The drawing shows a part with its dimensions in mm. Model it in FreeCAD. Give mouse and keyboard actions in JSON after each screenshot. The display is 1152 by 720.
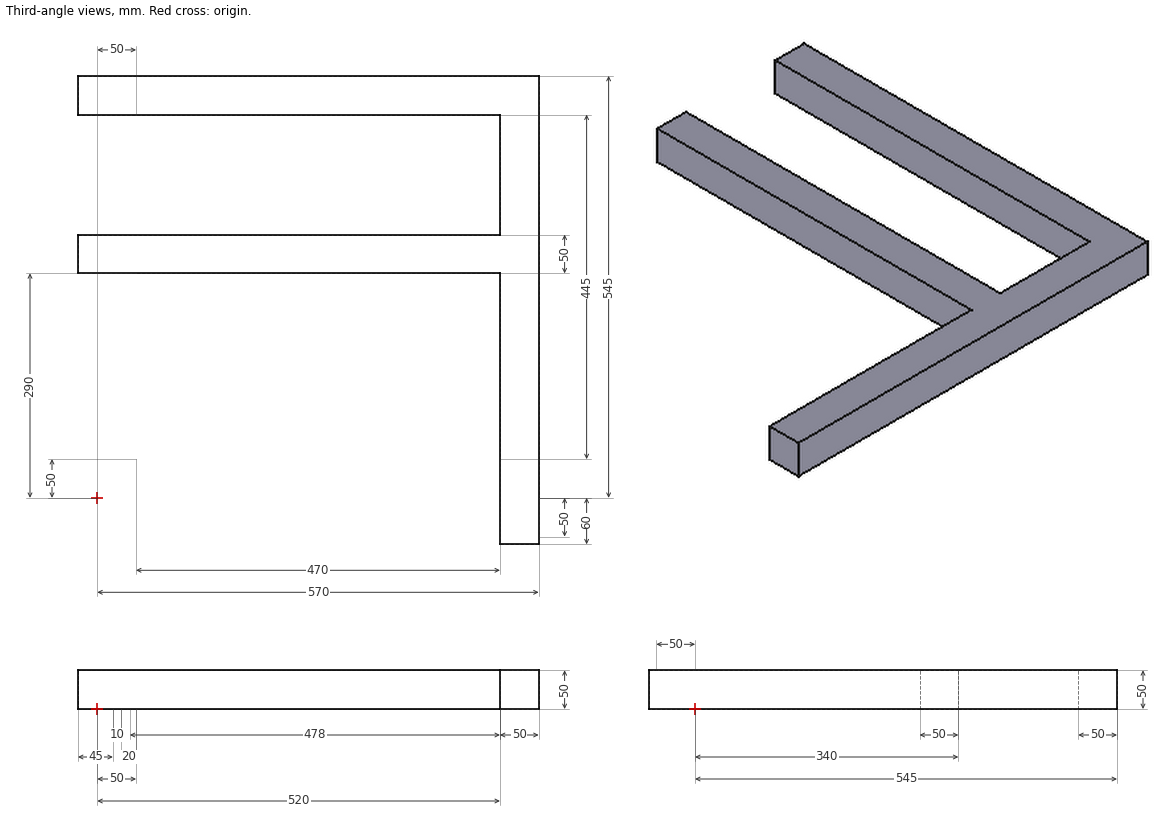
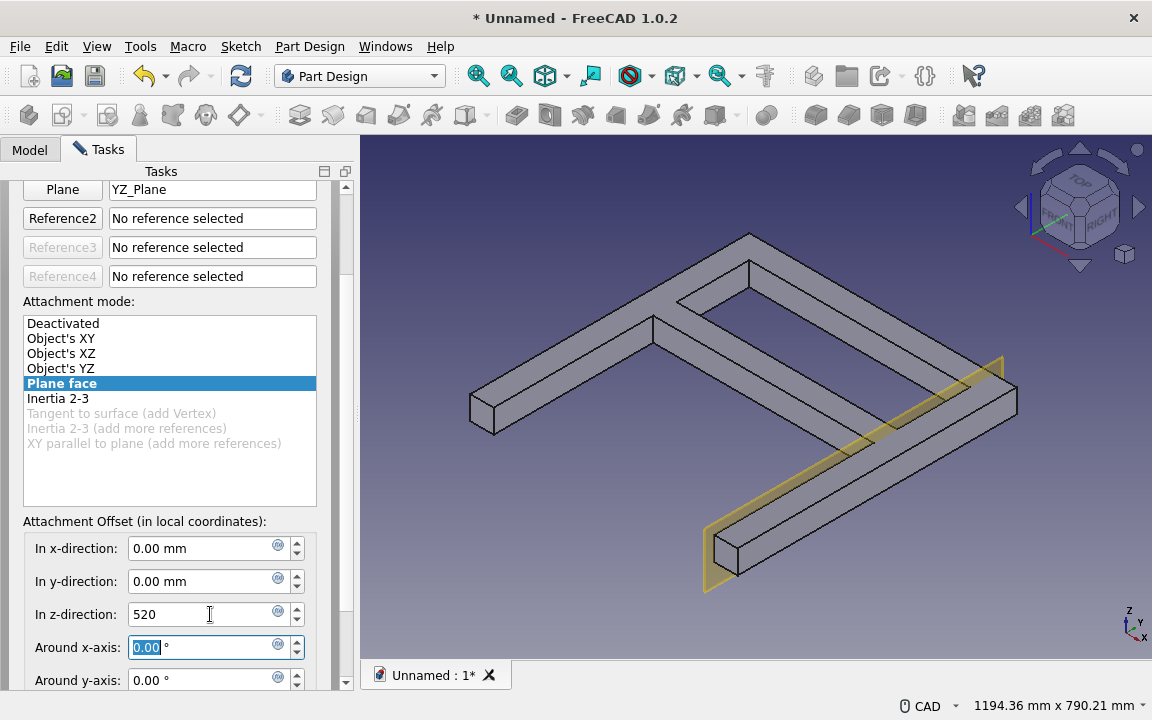
{"action": "scroll", "coordinate": [346, 436], "scroll_direction": "up", "scroll_amount": 3}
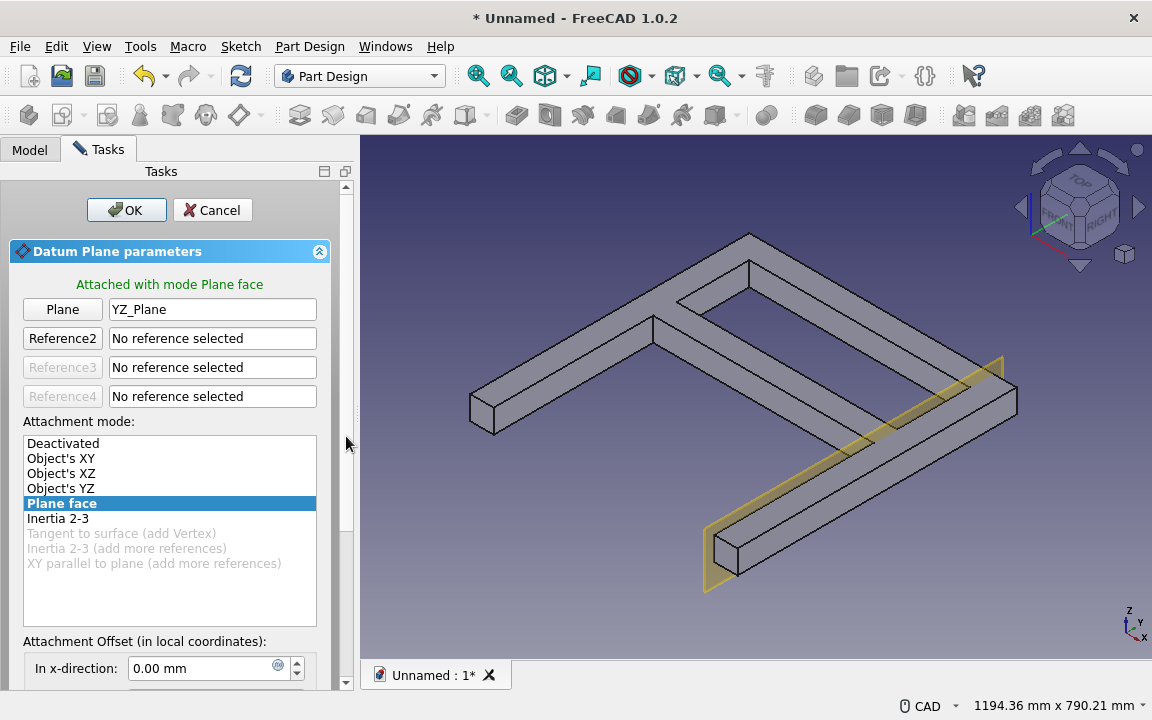
{"action": "left_click", "coordinate": [127, 210]}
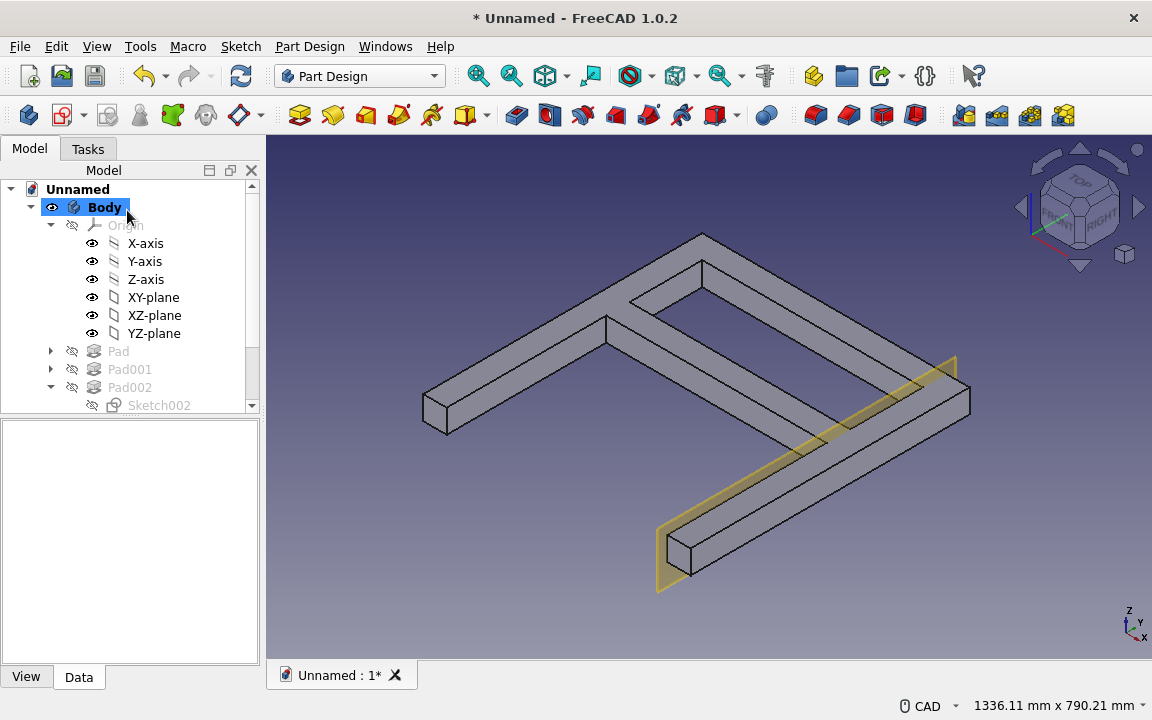
{"action": "scroll", "coordinate": [101, 293], "scroll_direction": "down", "scroll_amount": 3}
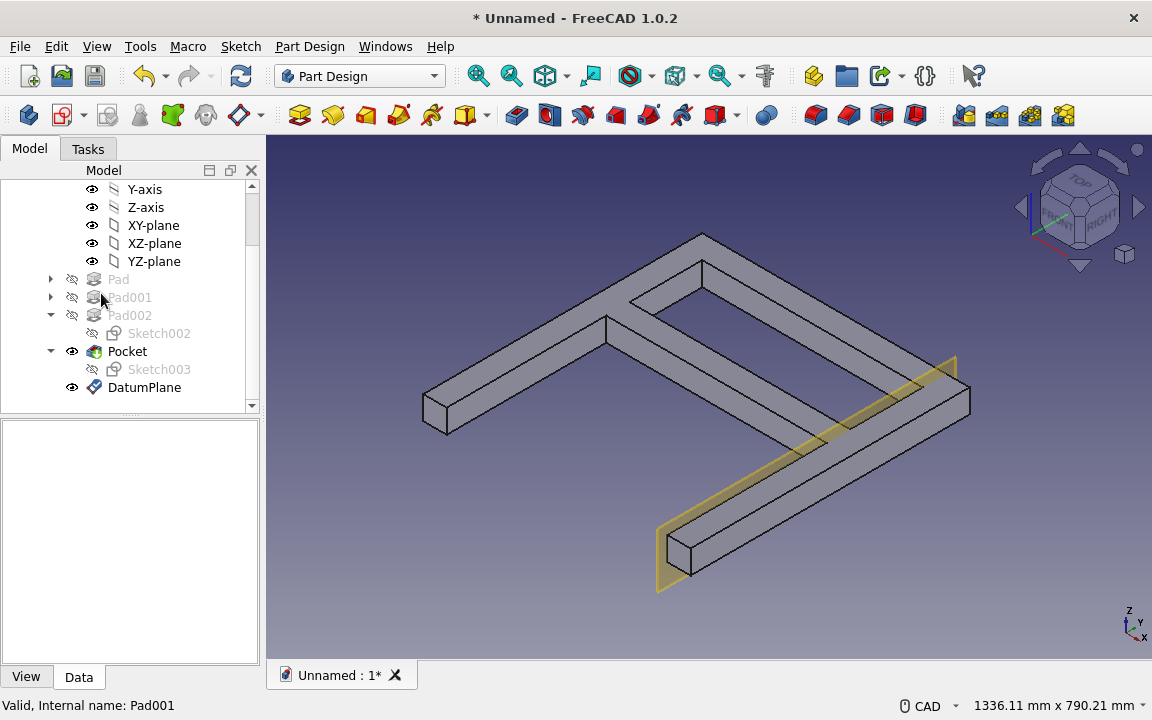
{"action": "left_click", "coordinate": [117, 387]}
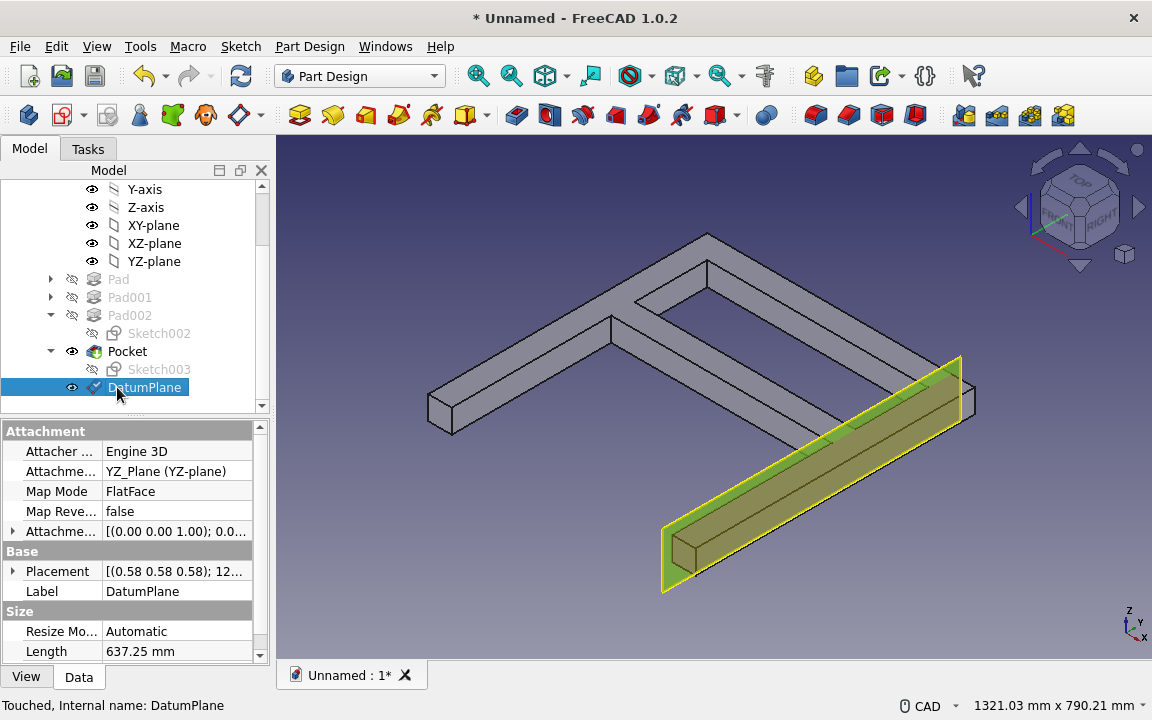
{"action": "left_click", "coordinate": [62, 116]}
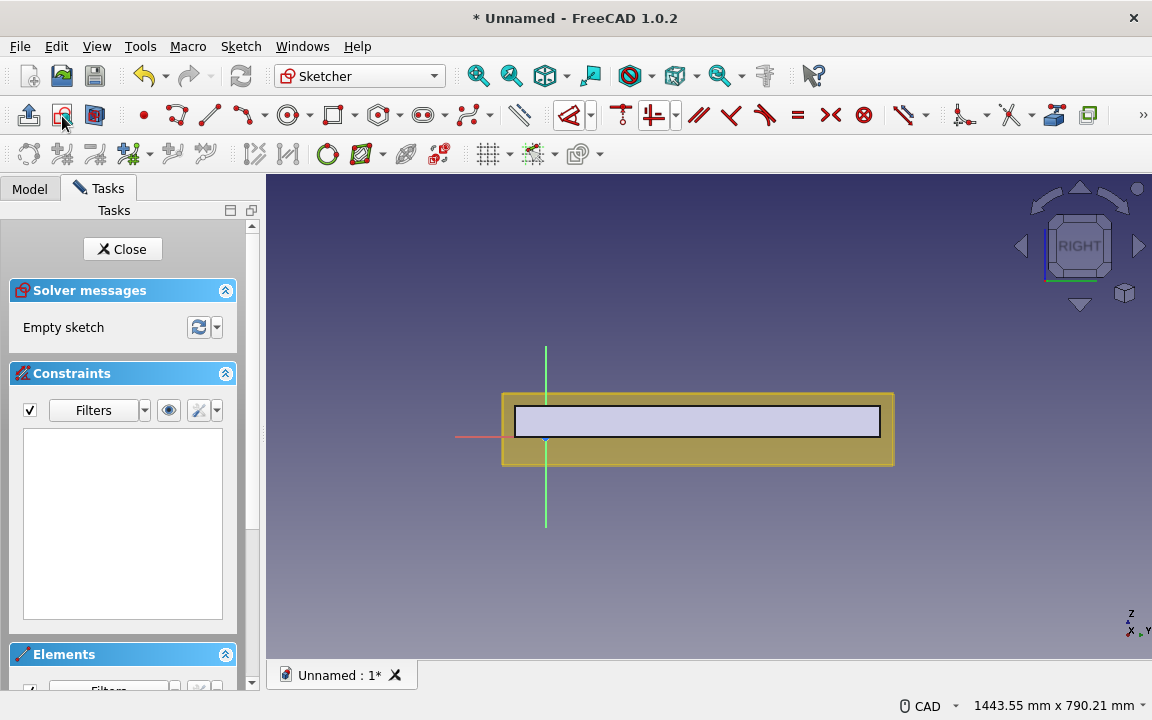
{"action": "key", "text": "q s"}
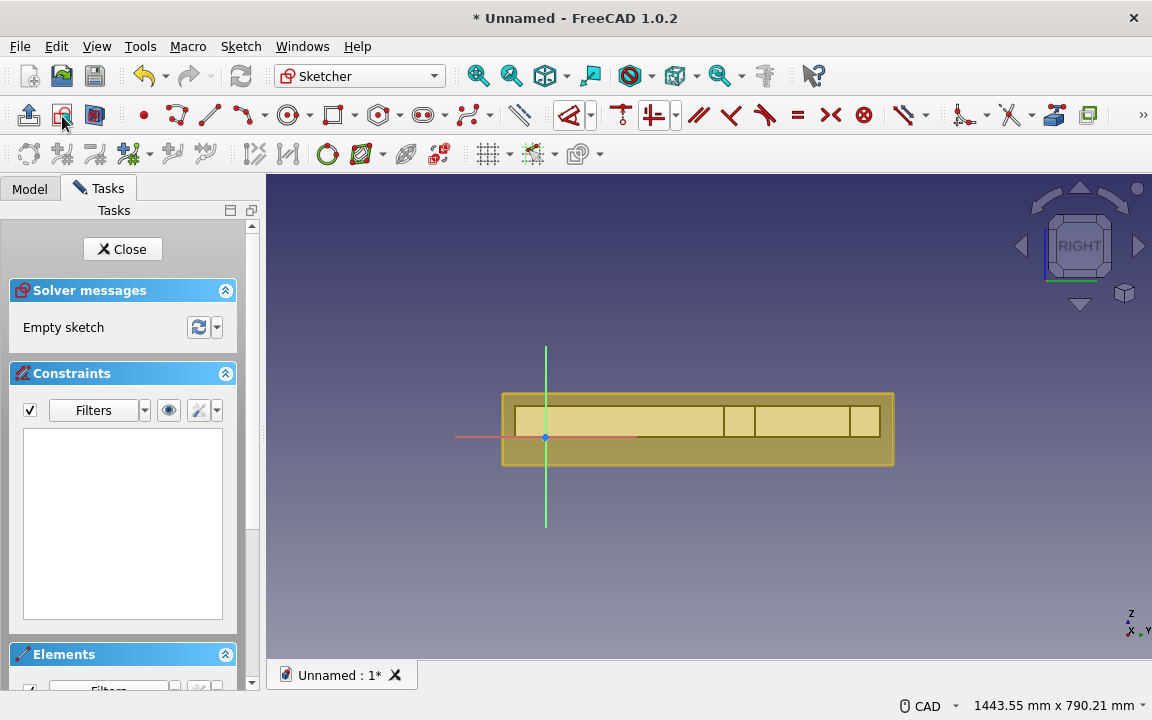
{"action": "scroll", "coordinate": [517, 422], "scroll_direction": "up", "scroll_amount": 11}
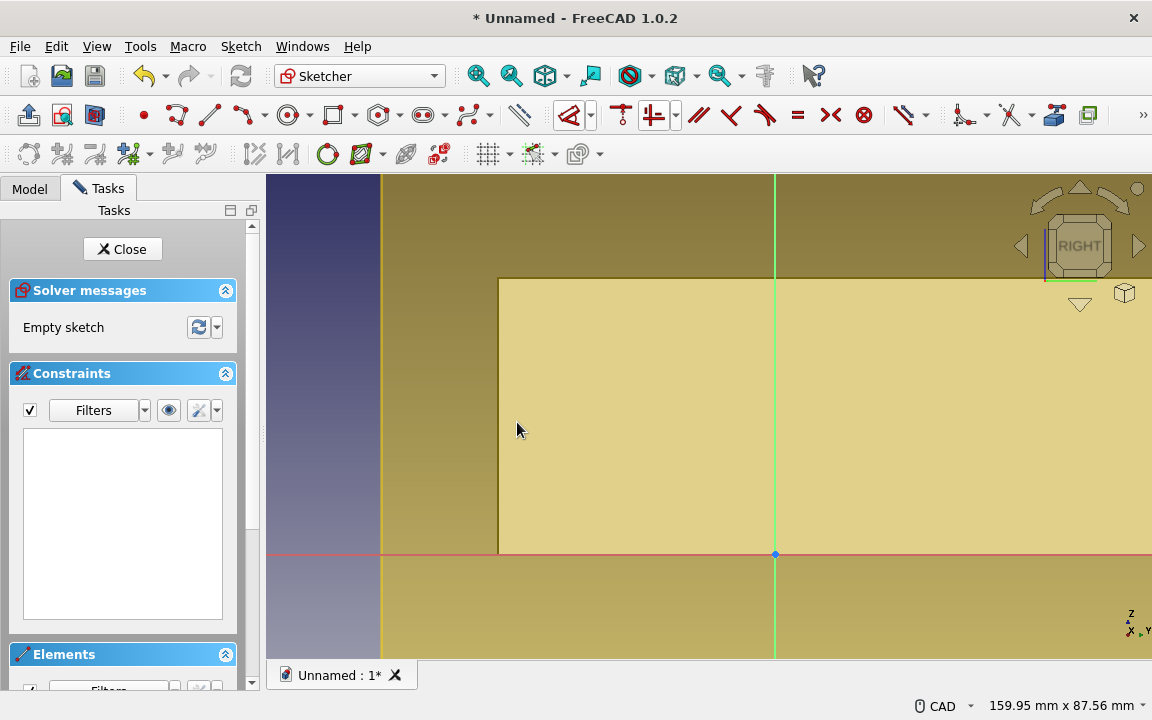
{"action": "key", "text": "g r"}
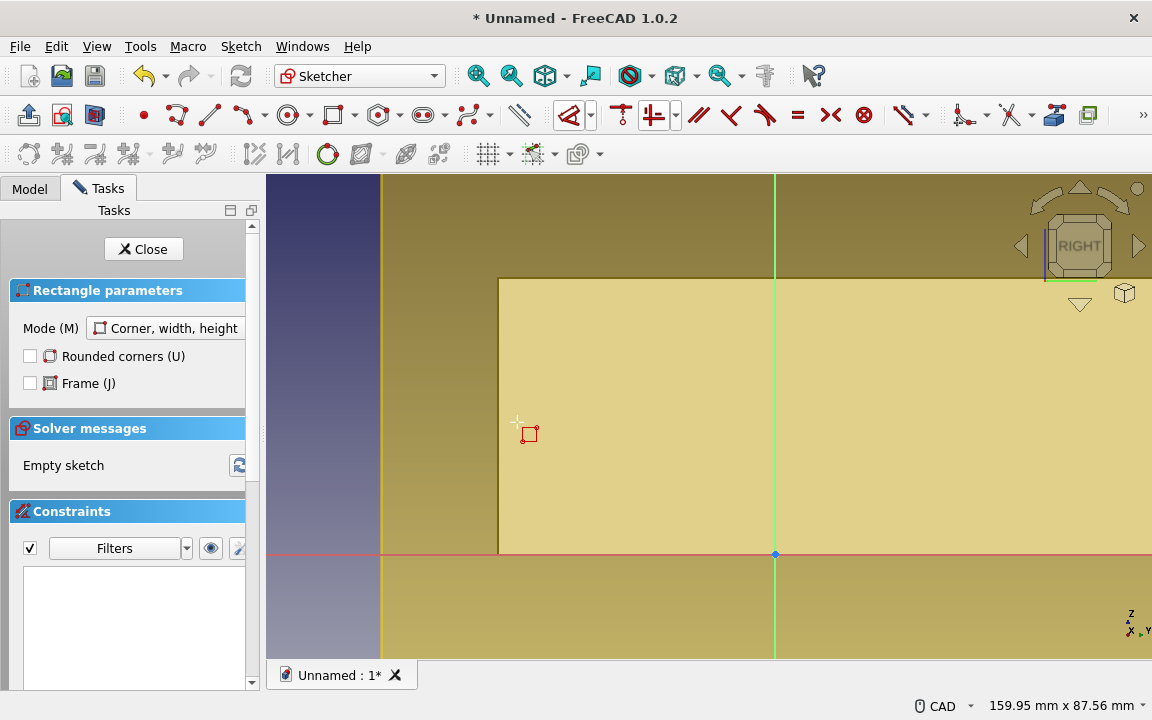
{"action": "left_click", "coordinate": [775, 555]}
{"action": "mouse_move", "coordinate": [498, 278]}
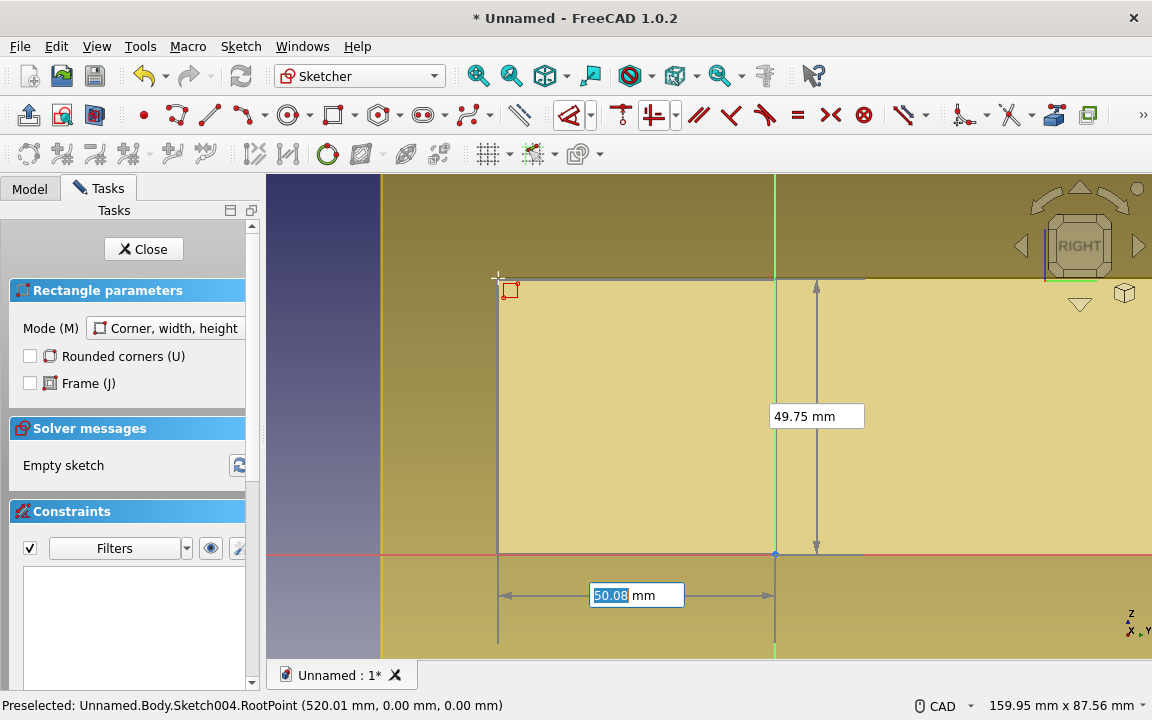
{"action": "type", "text": "50"}
{"action": "key", "text": "Tab"}
{"action": "type", "text": "50"}
{"action": "key", "text": "Return"}
{"action": "key", "text": "Escape"}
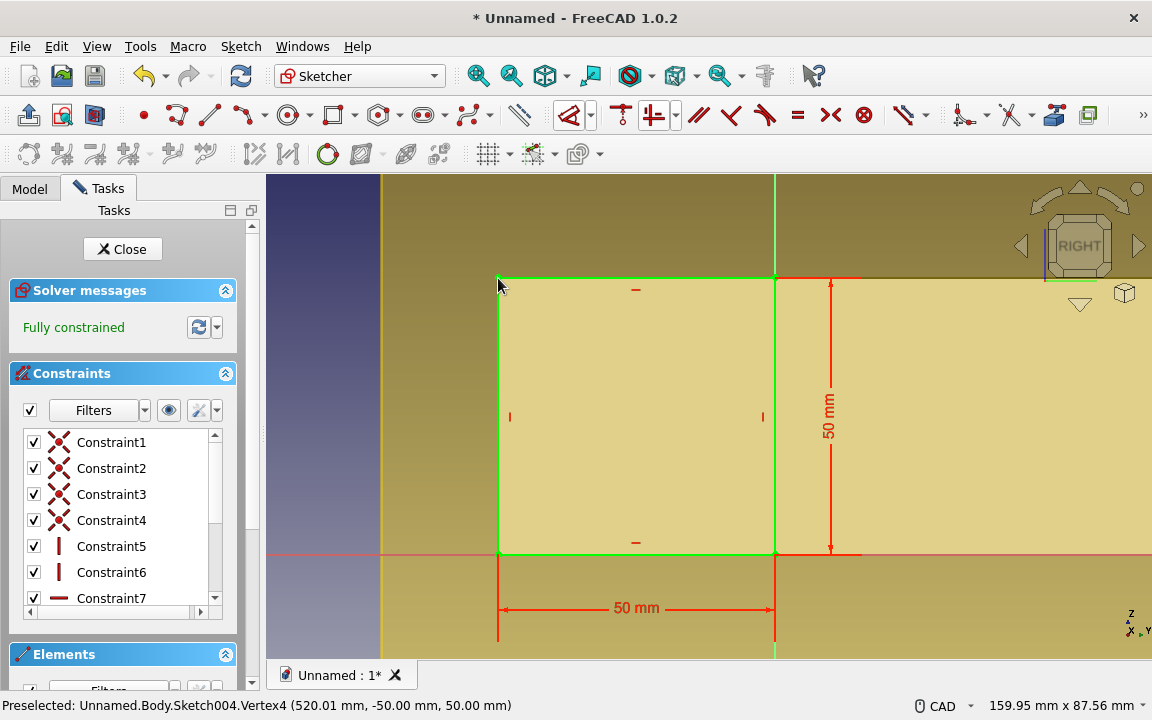
{"action": "left_click", "coordinate": [123, 249]}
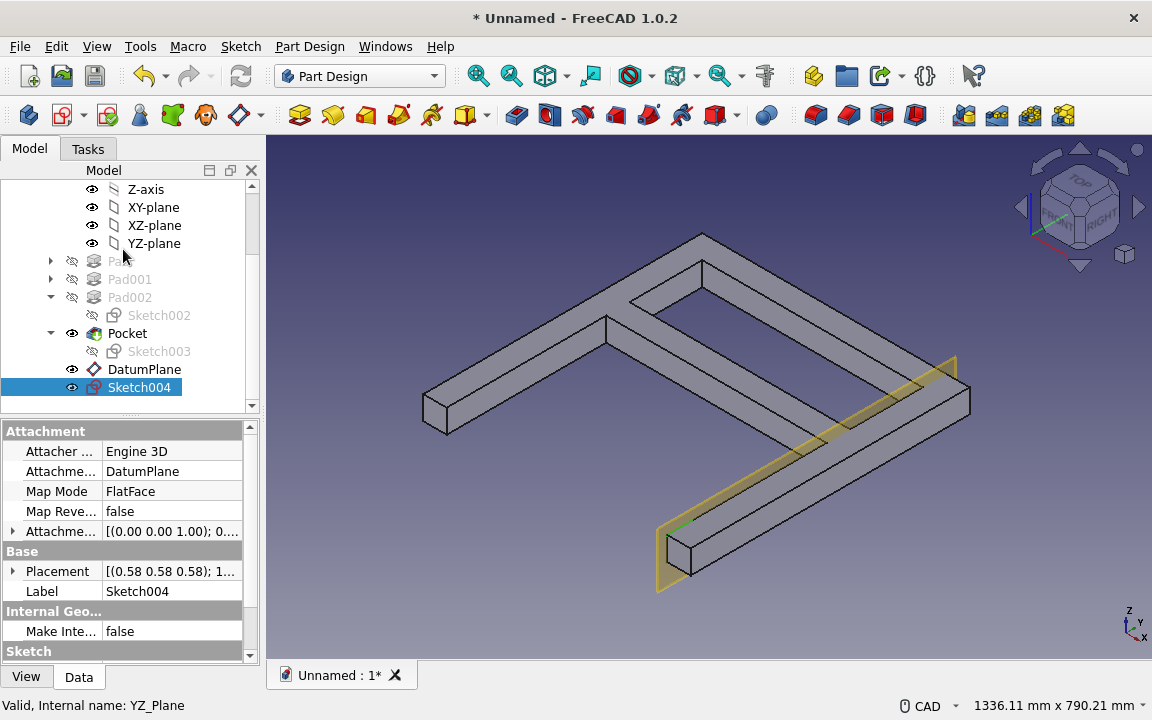
{"action": "left_click", "coordinate": [300, 116]}